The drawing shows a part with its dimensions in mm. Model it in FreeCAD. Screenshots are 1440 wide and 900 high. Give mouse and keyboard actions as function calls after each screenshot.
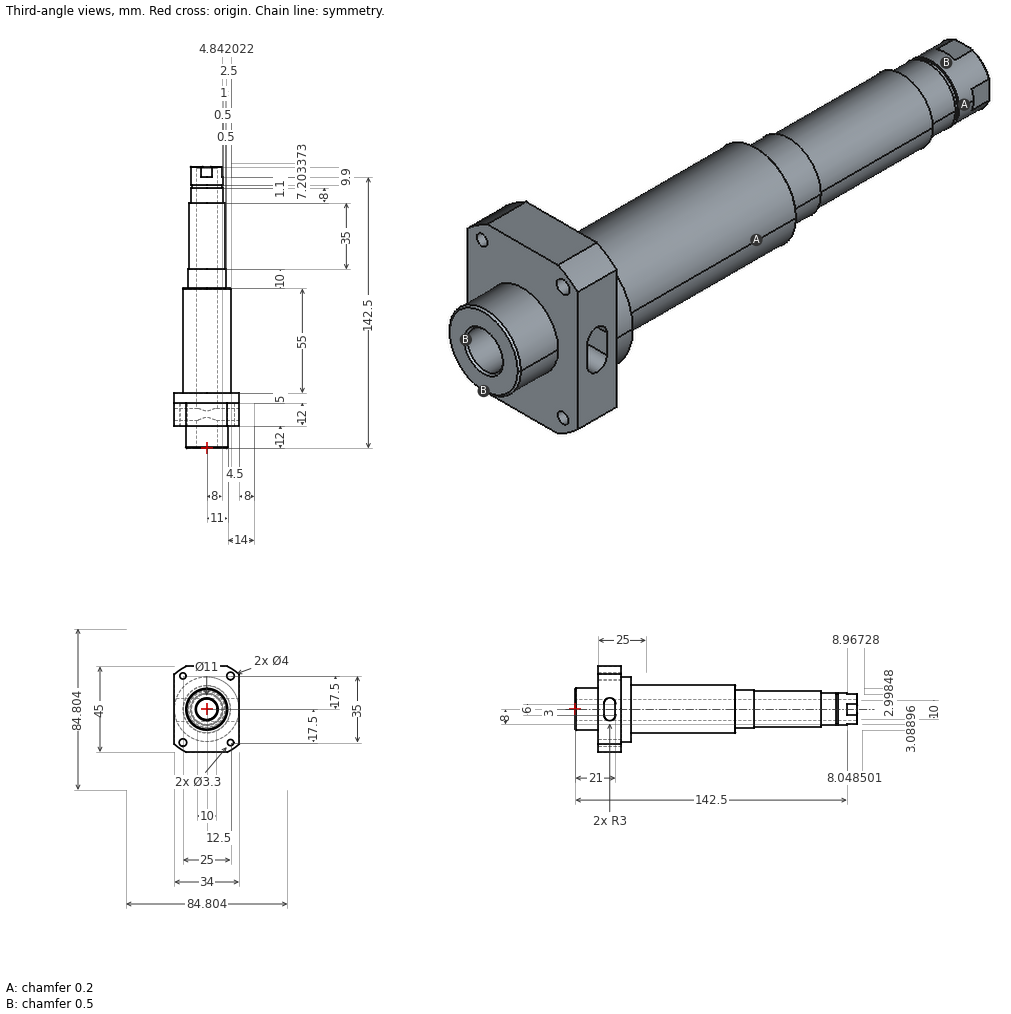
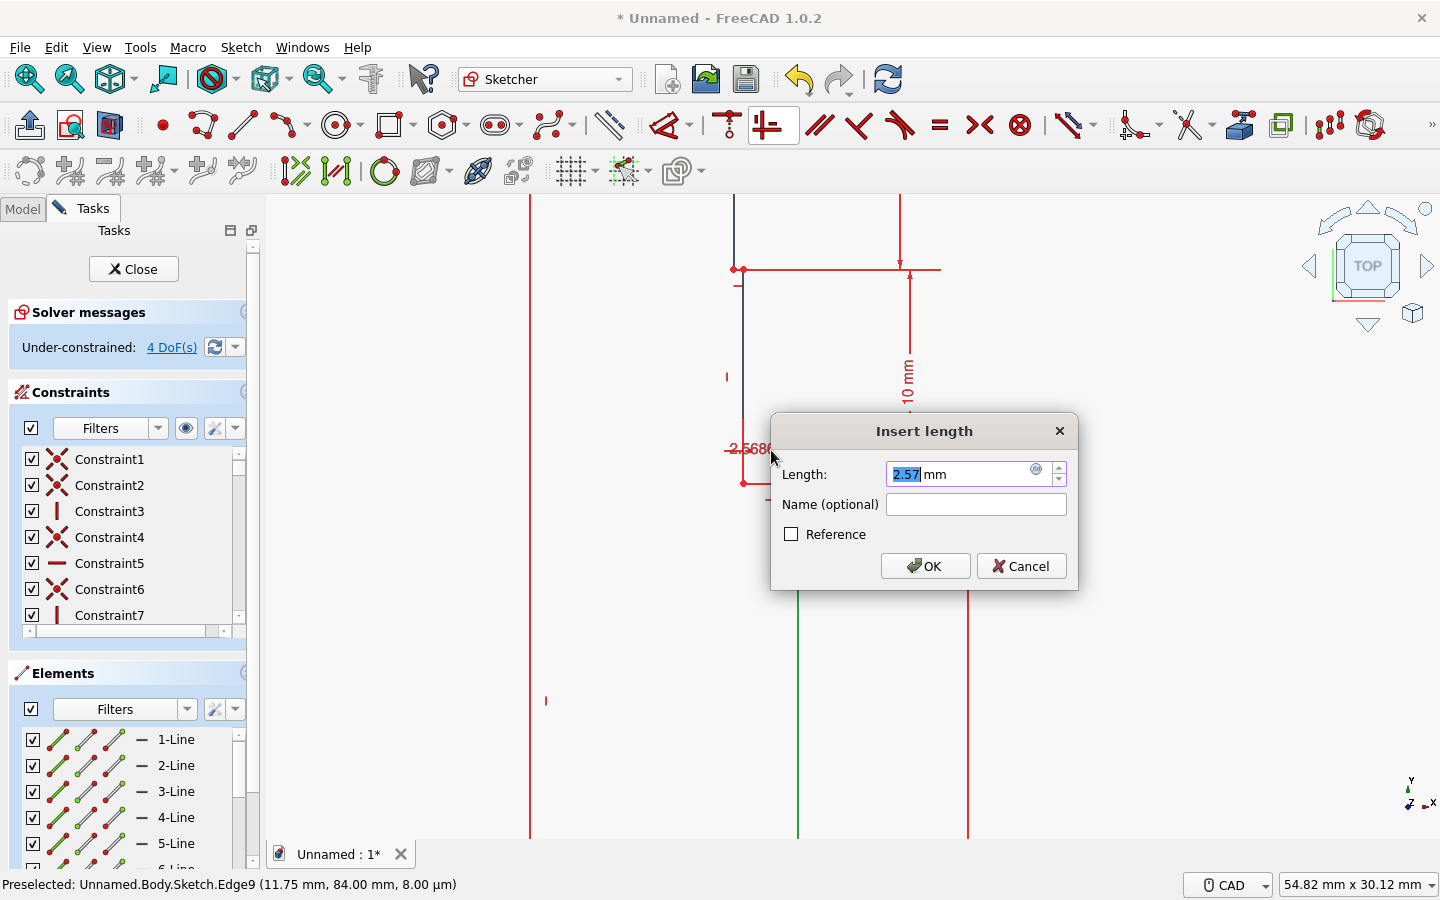
text(2.5)
key(Return)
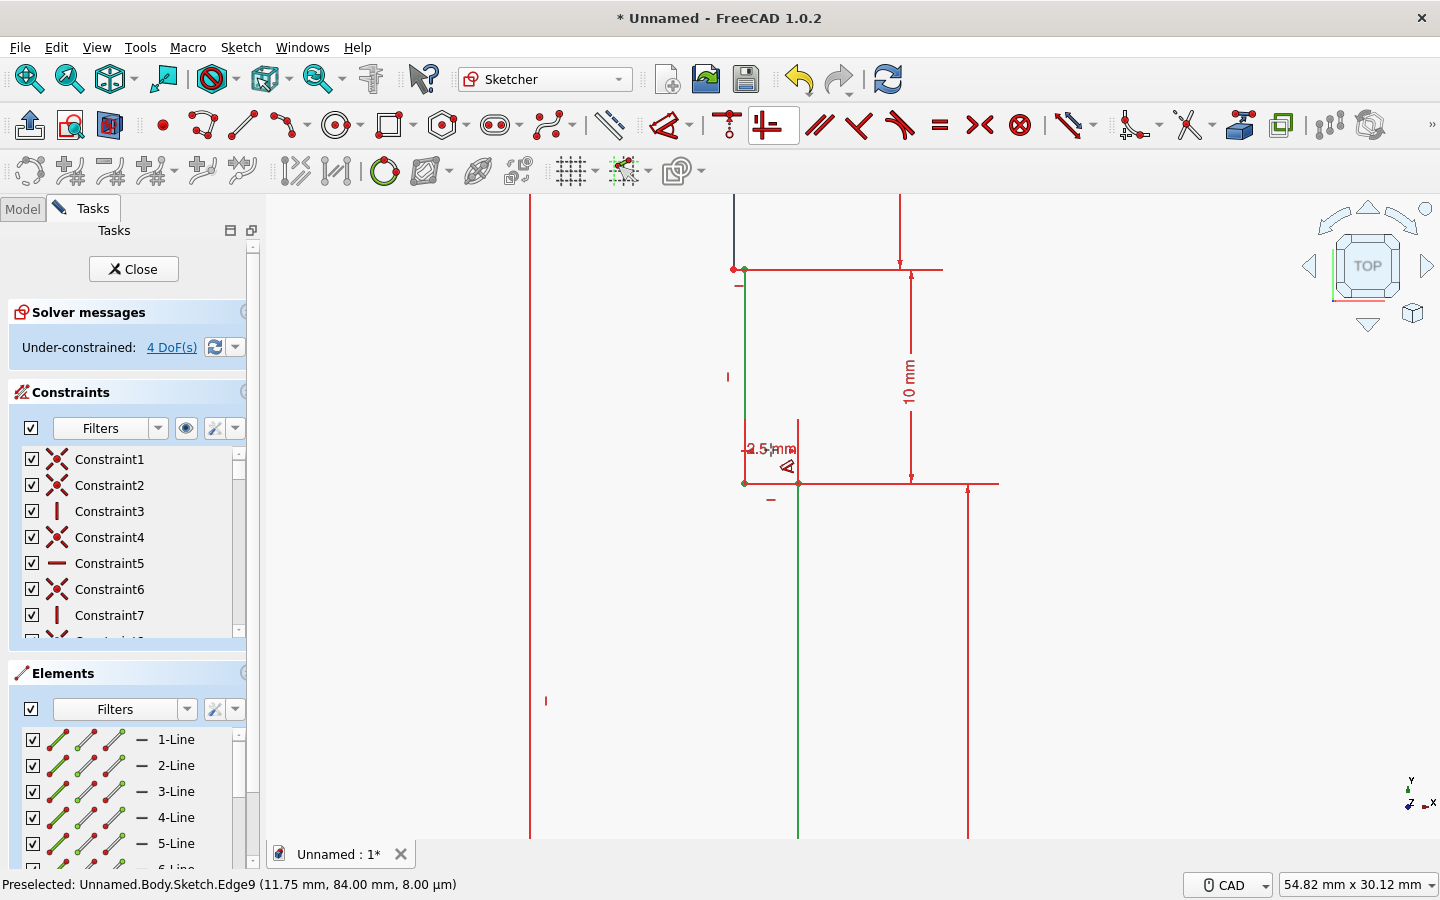
scroll(739, 270, up, 7)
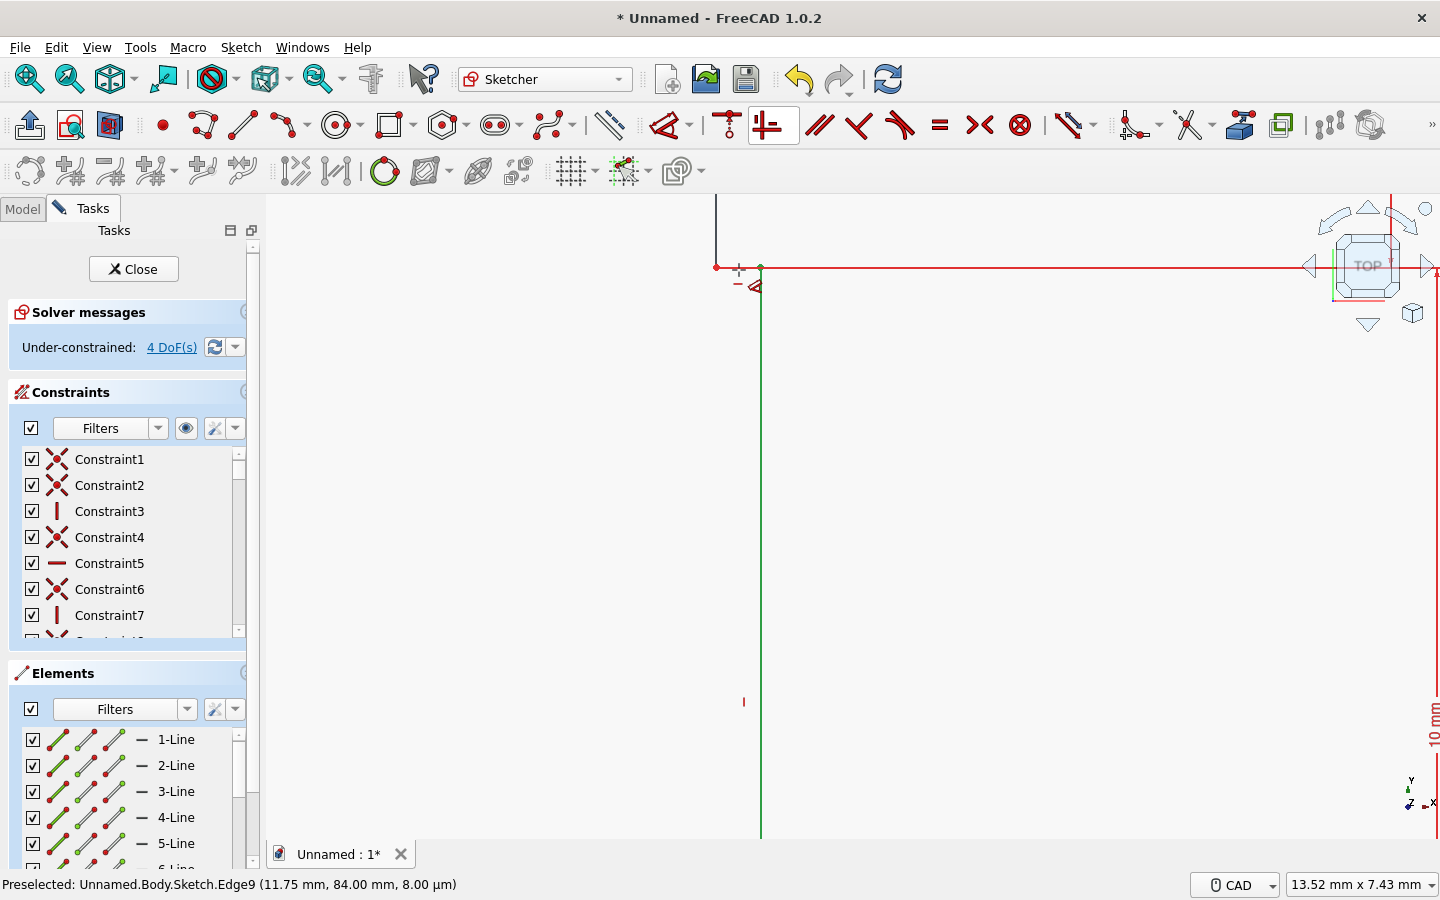
click(738, 268)
click(738, 234)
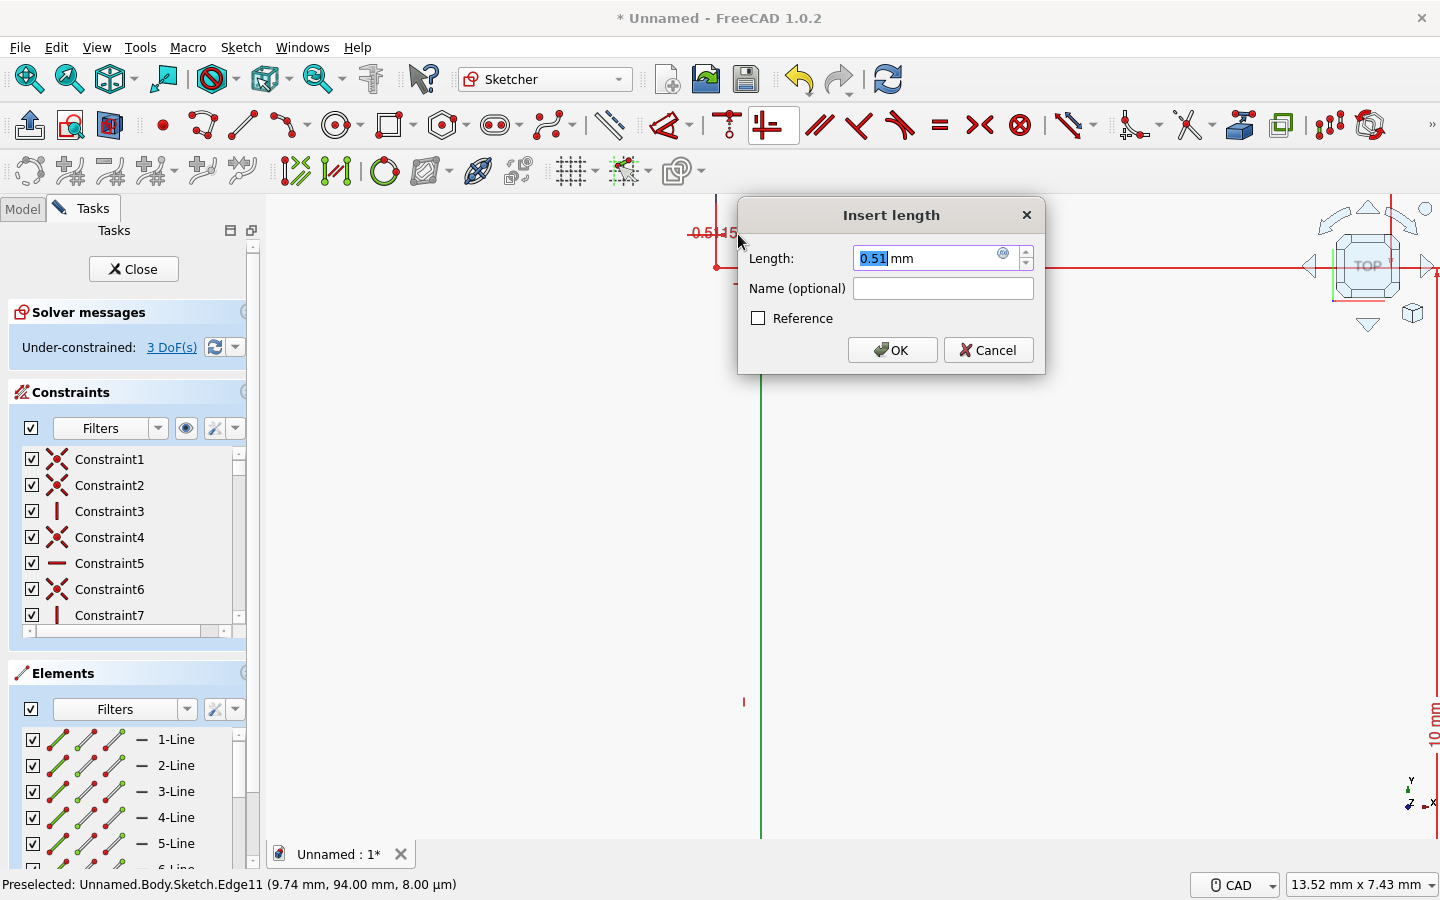
text(0.5)
key(Return)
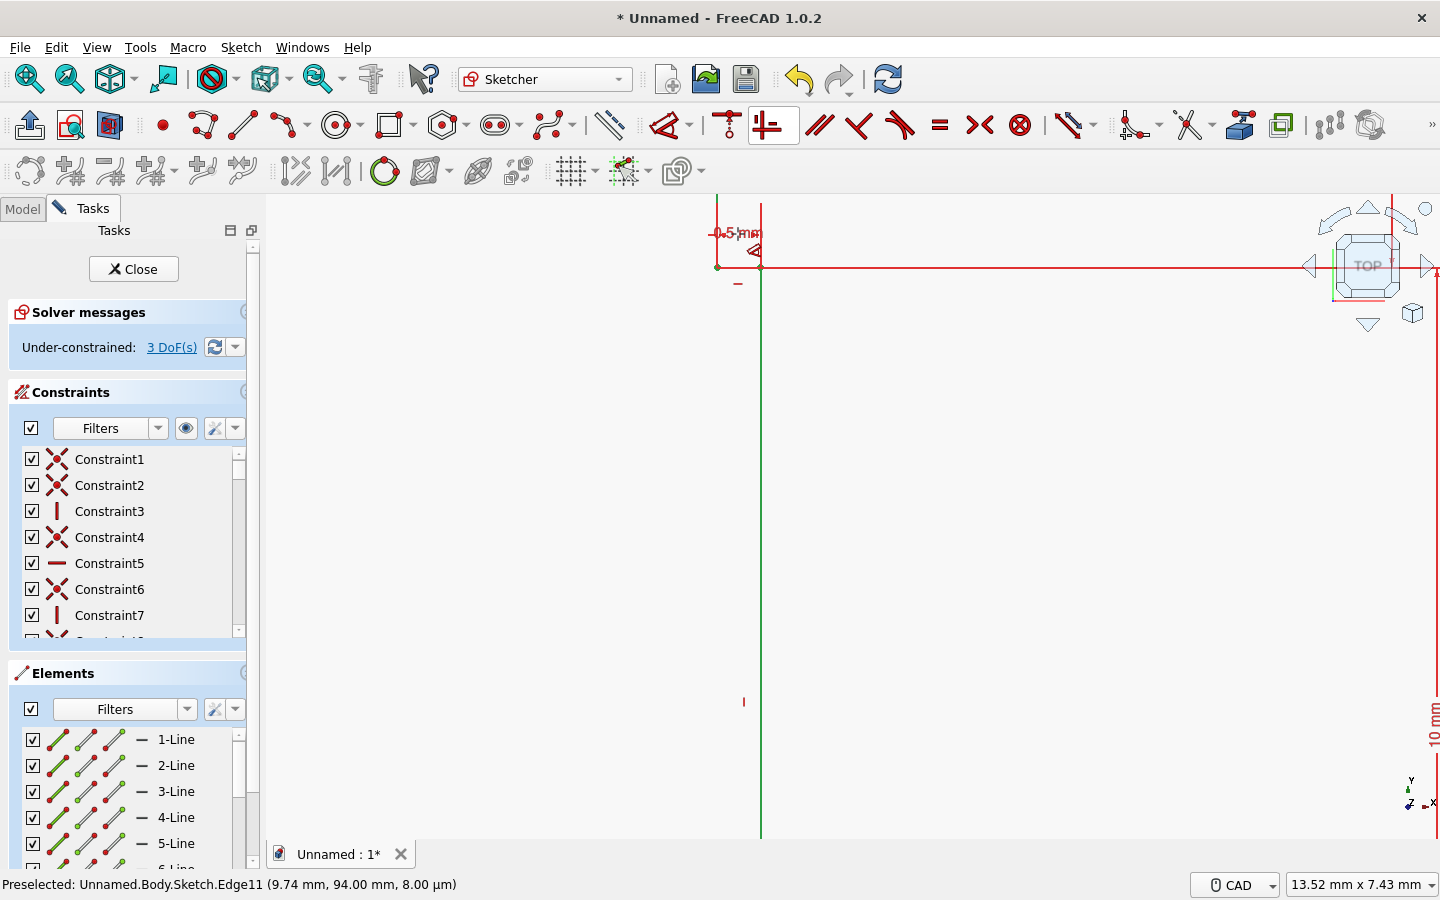
scroll(776, 453, down, 16)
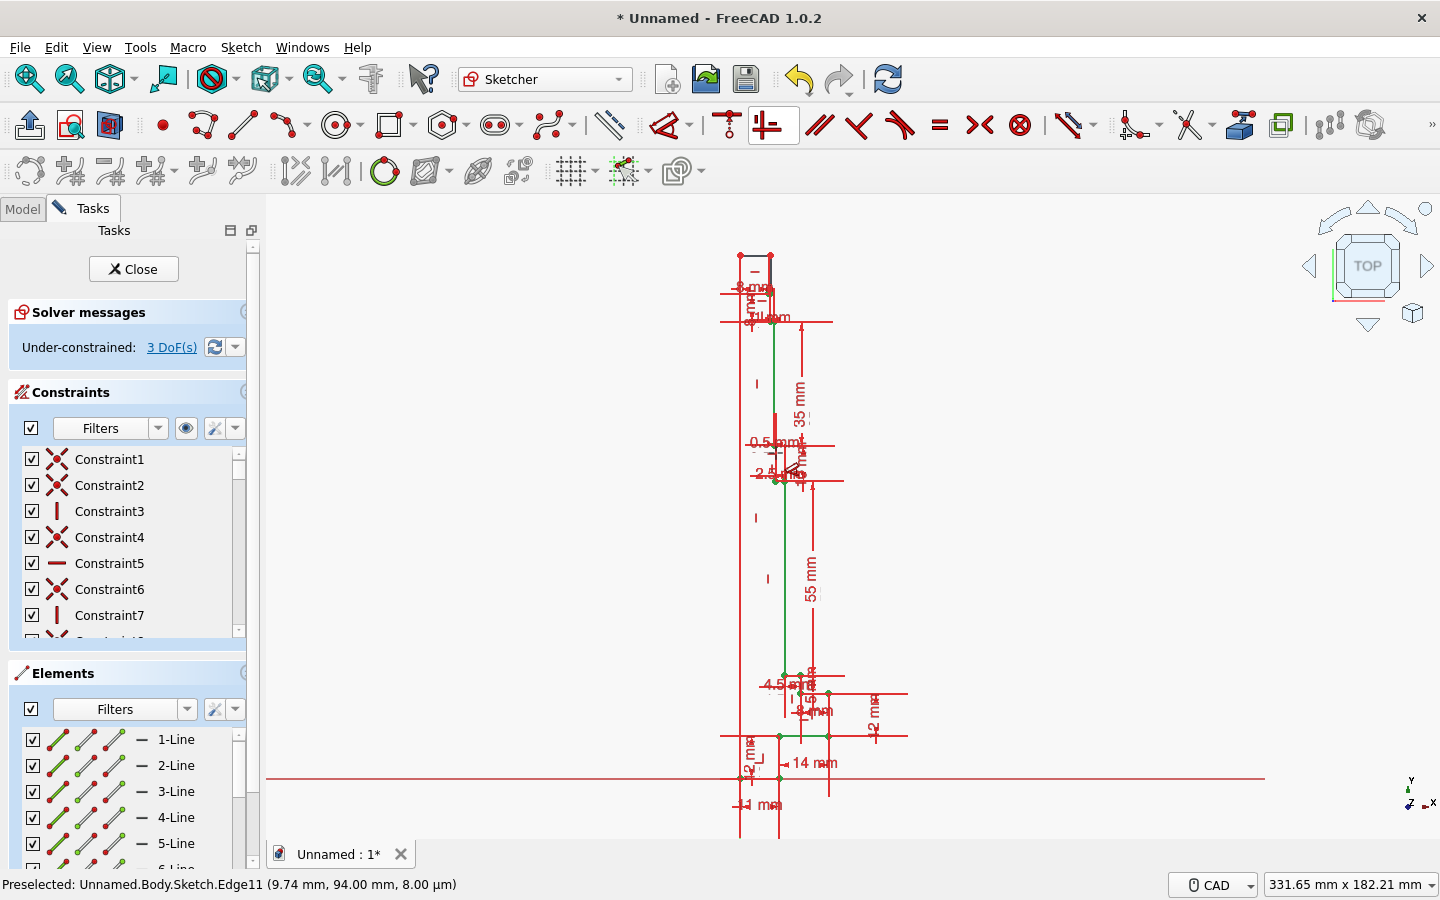
scroll(769, 292, up, 13)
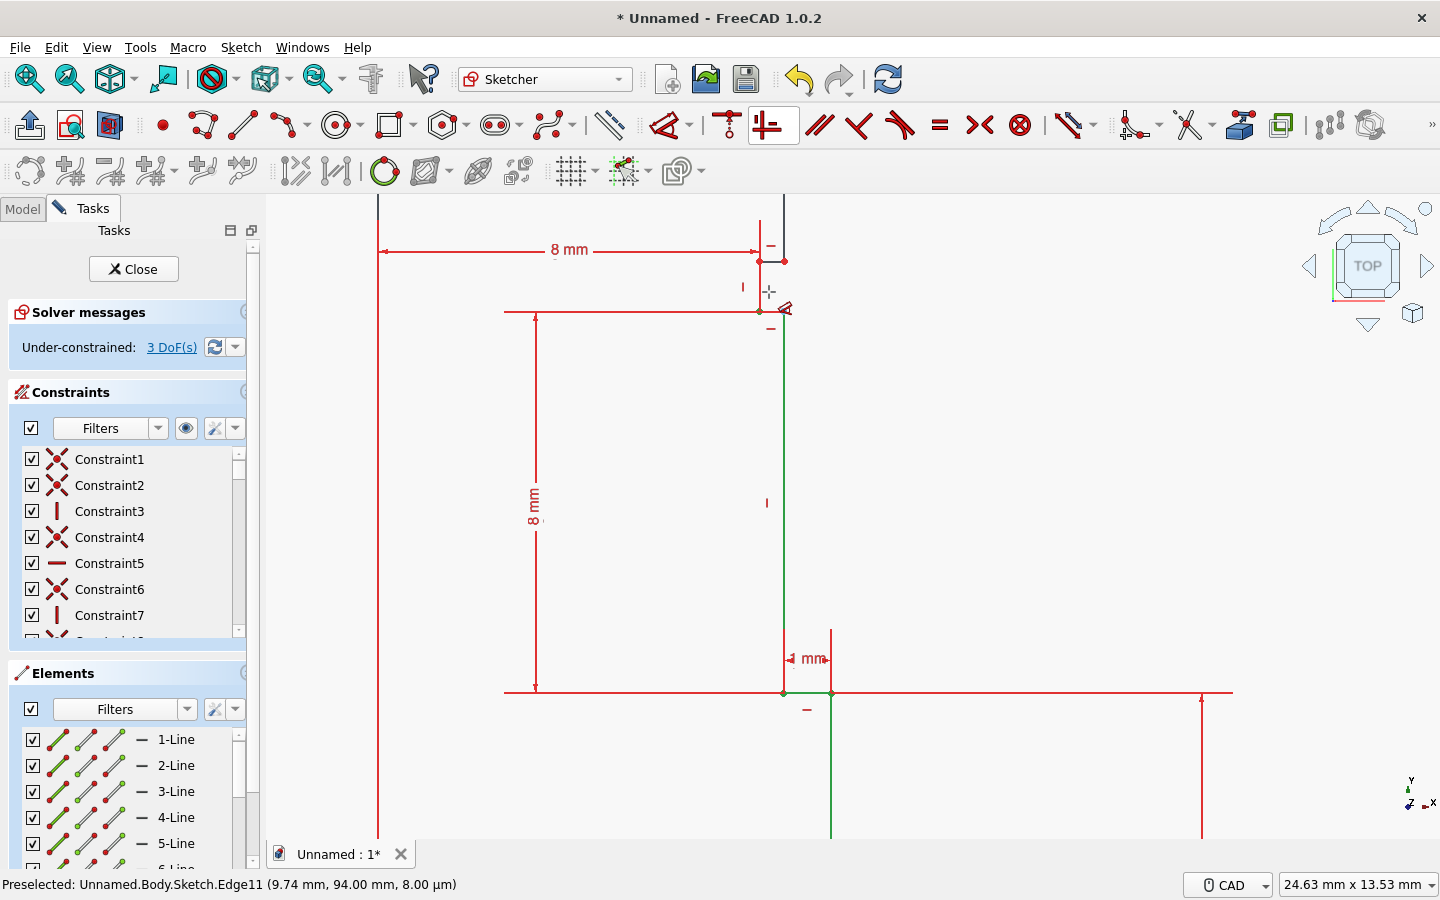
click(760, 297)
click(726, 287)